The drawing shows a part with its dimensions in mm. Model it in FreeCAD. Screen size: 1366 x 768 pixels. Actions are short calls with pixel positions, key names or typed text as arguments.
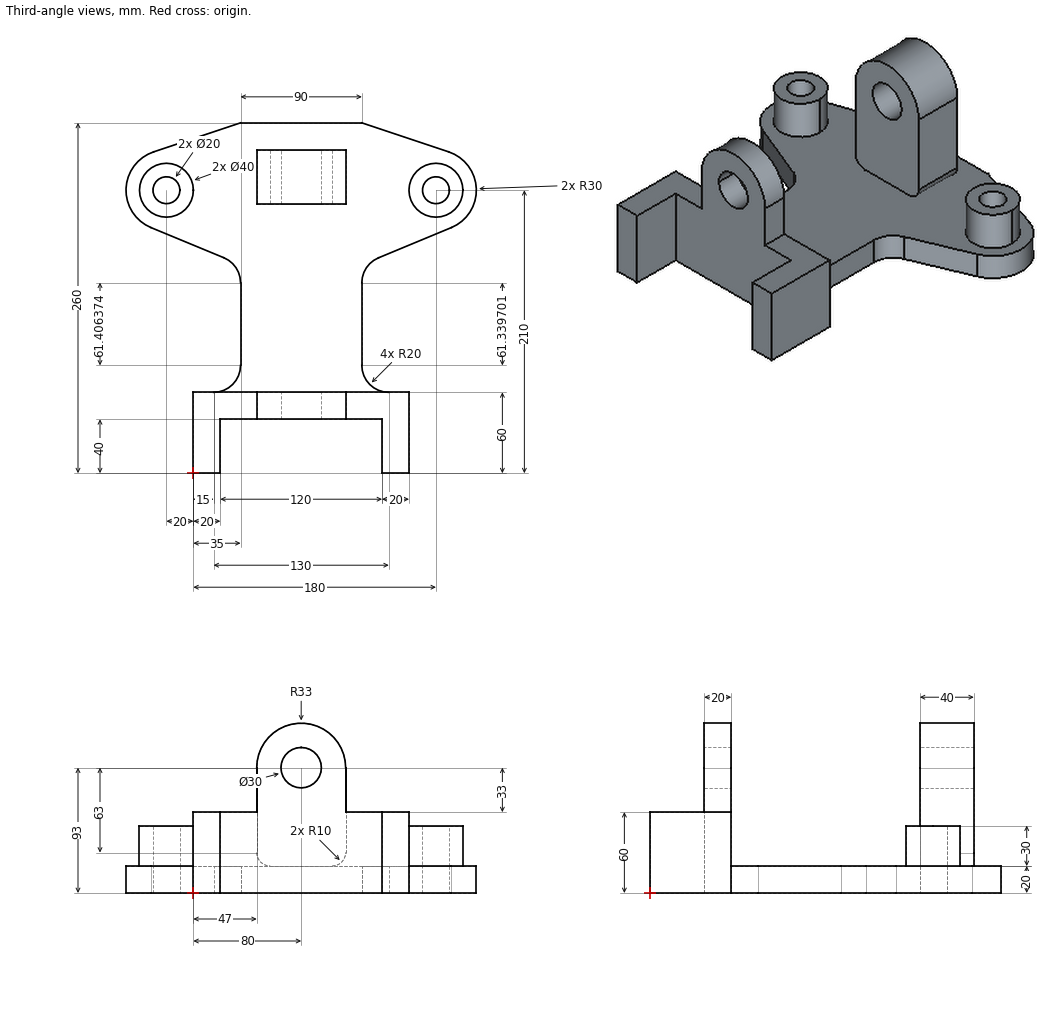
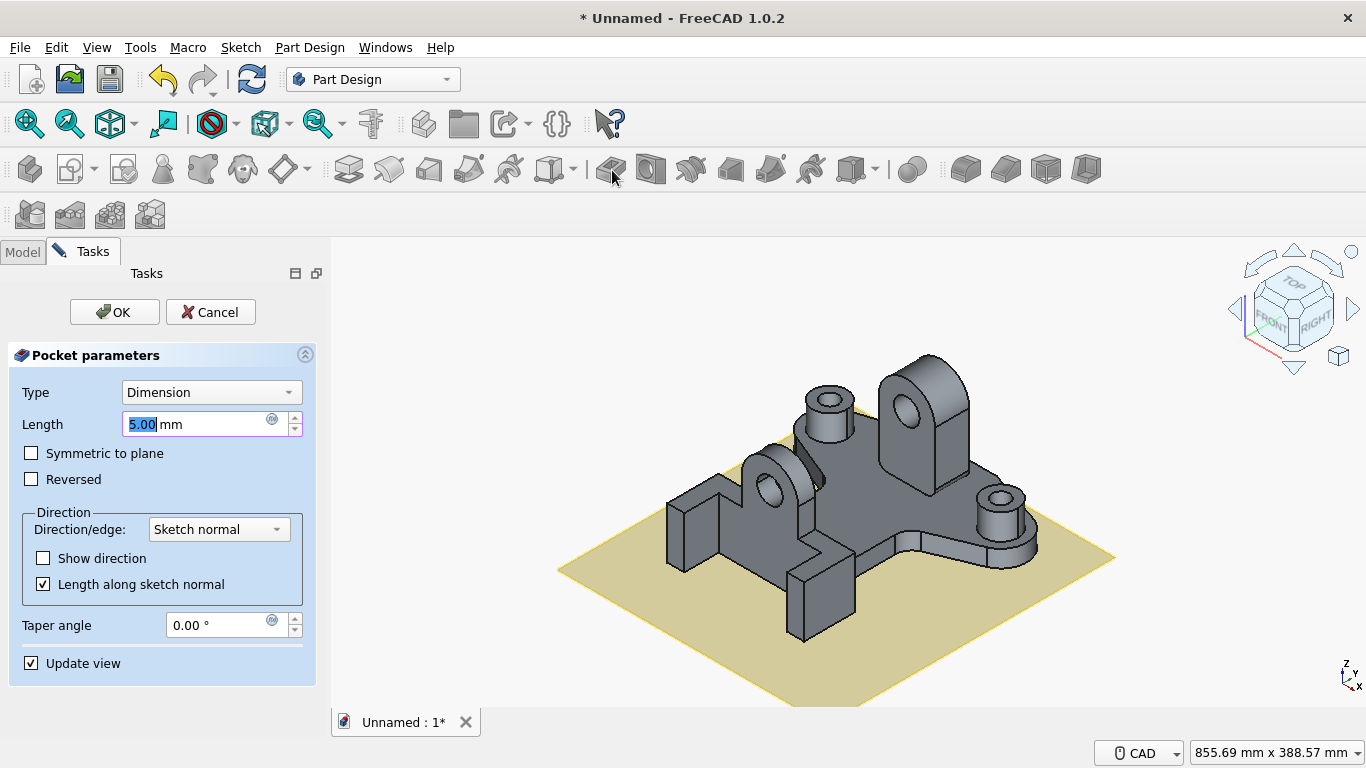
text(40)
key(Tab)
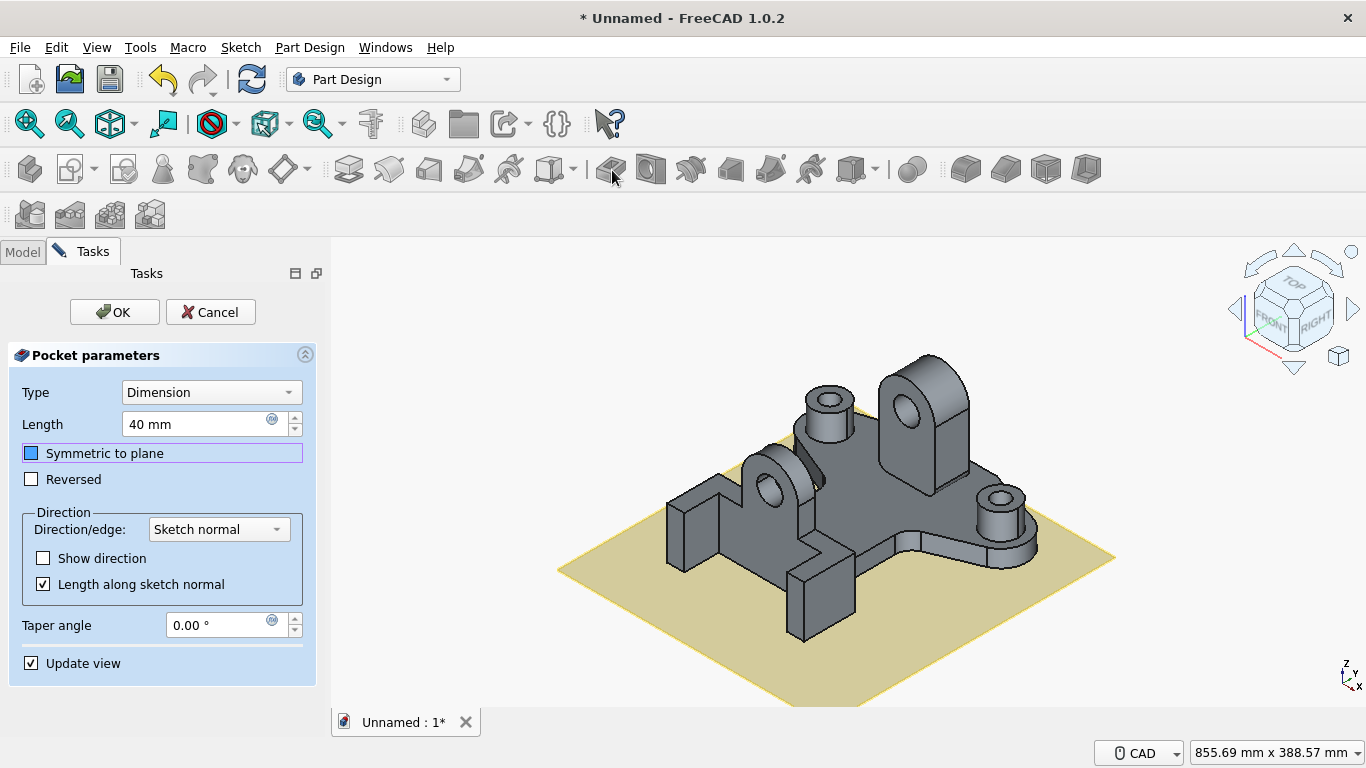
click(30, 479)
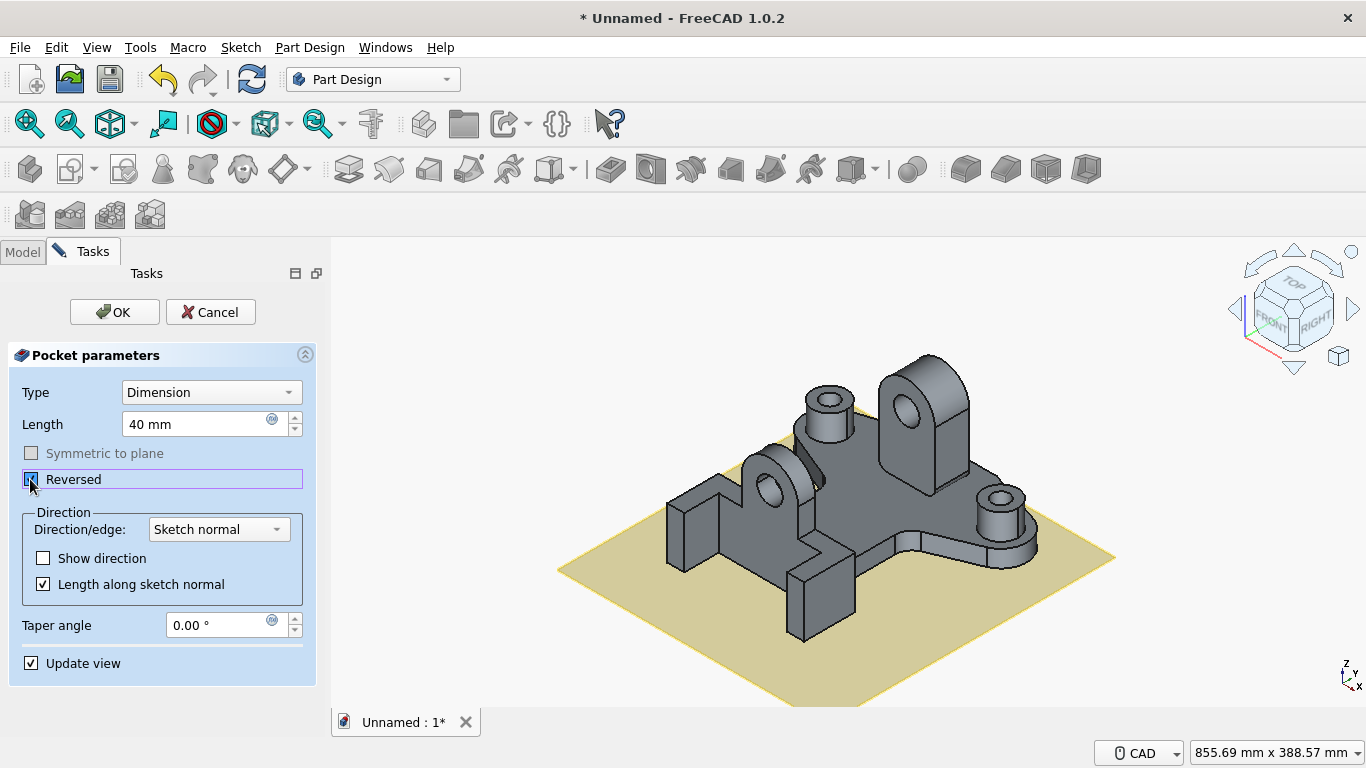
click(115, 312)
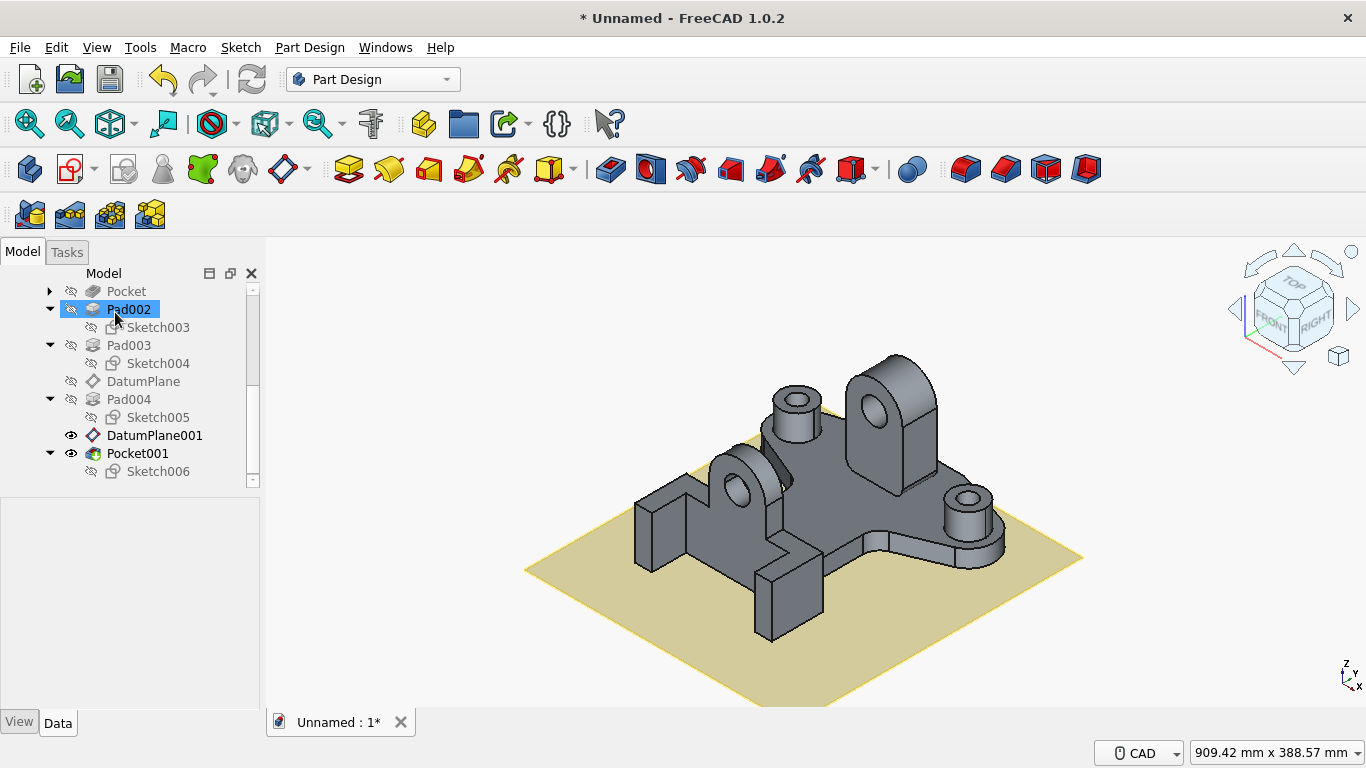
click(116, 435)
key(space)